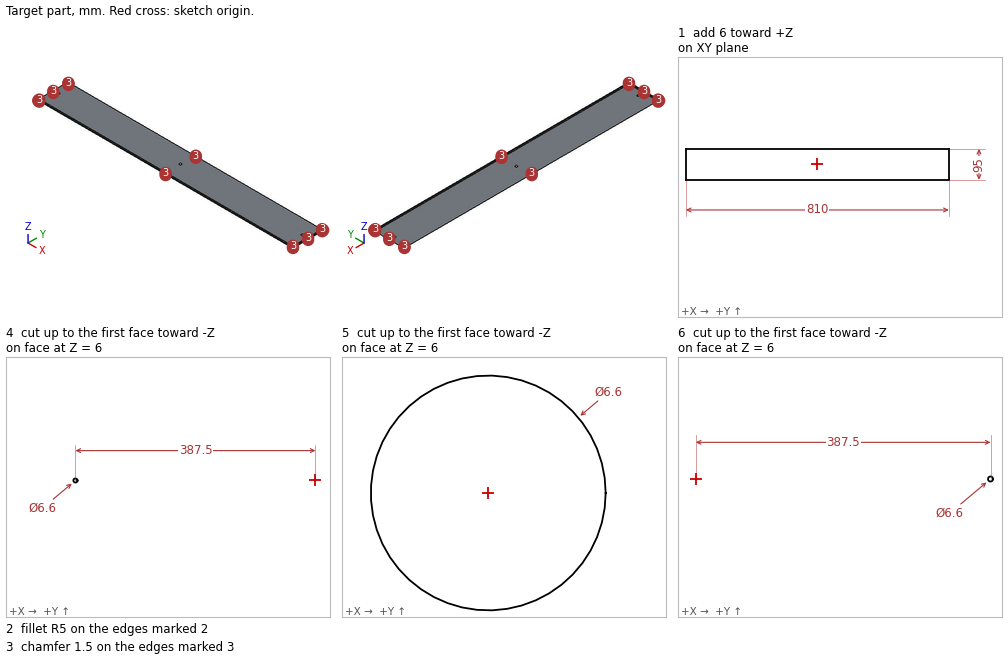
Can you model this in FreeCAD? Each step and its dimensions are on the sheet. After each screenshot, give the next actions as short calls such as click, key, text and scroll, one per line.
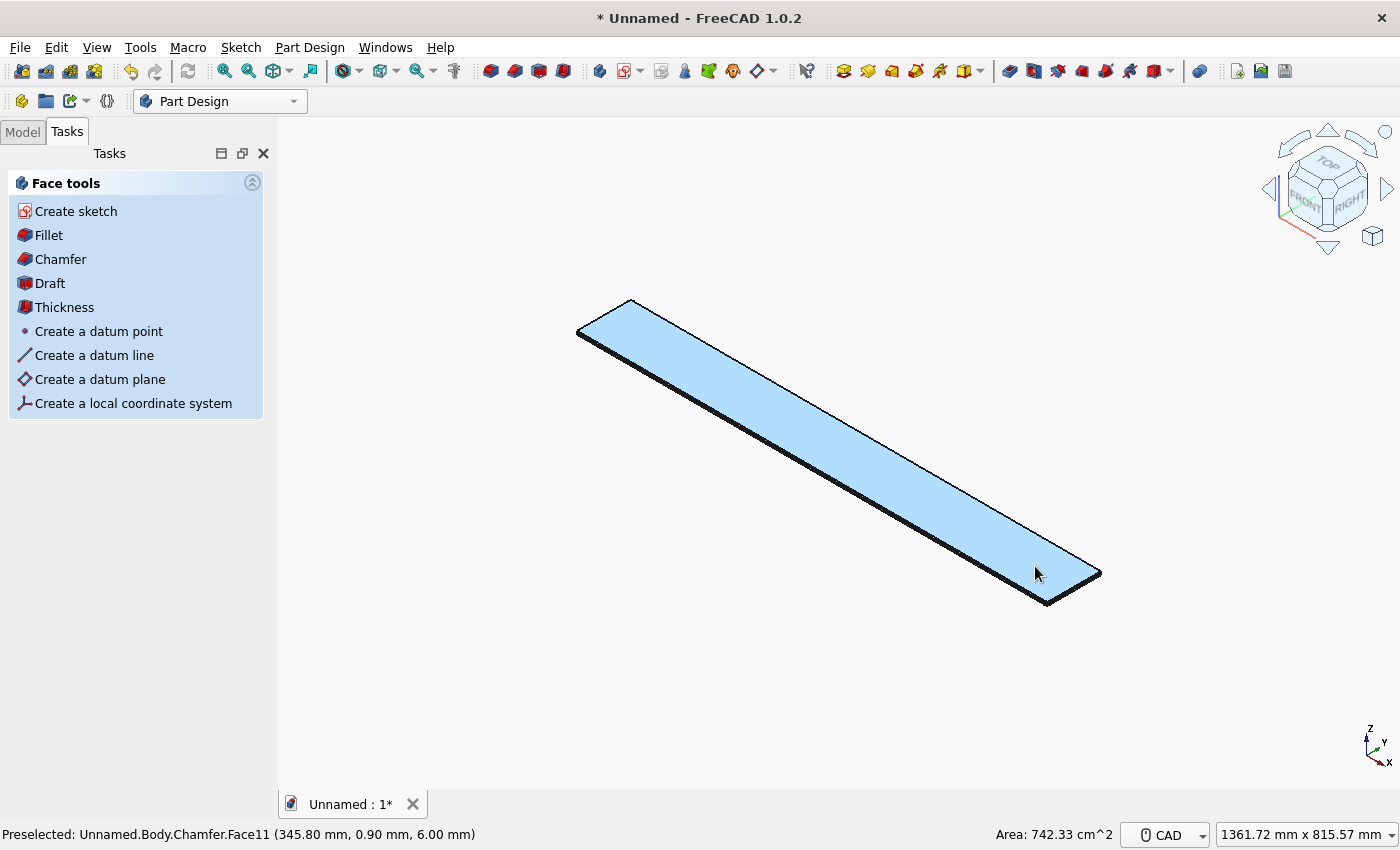
click(624, 72)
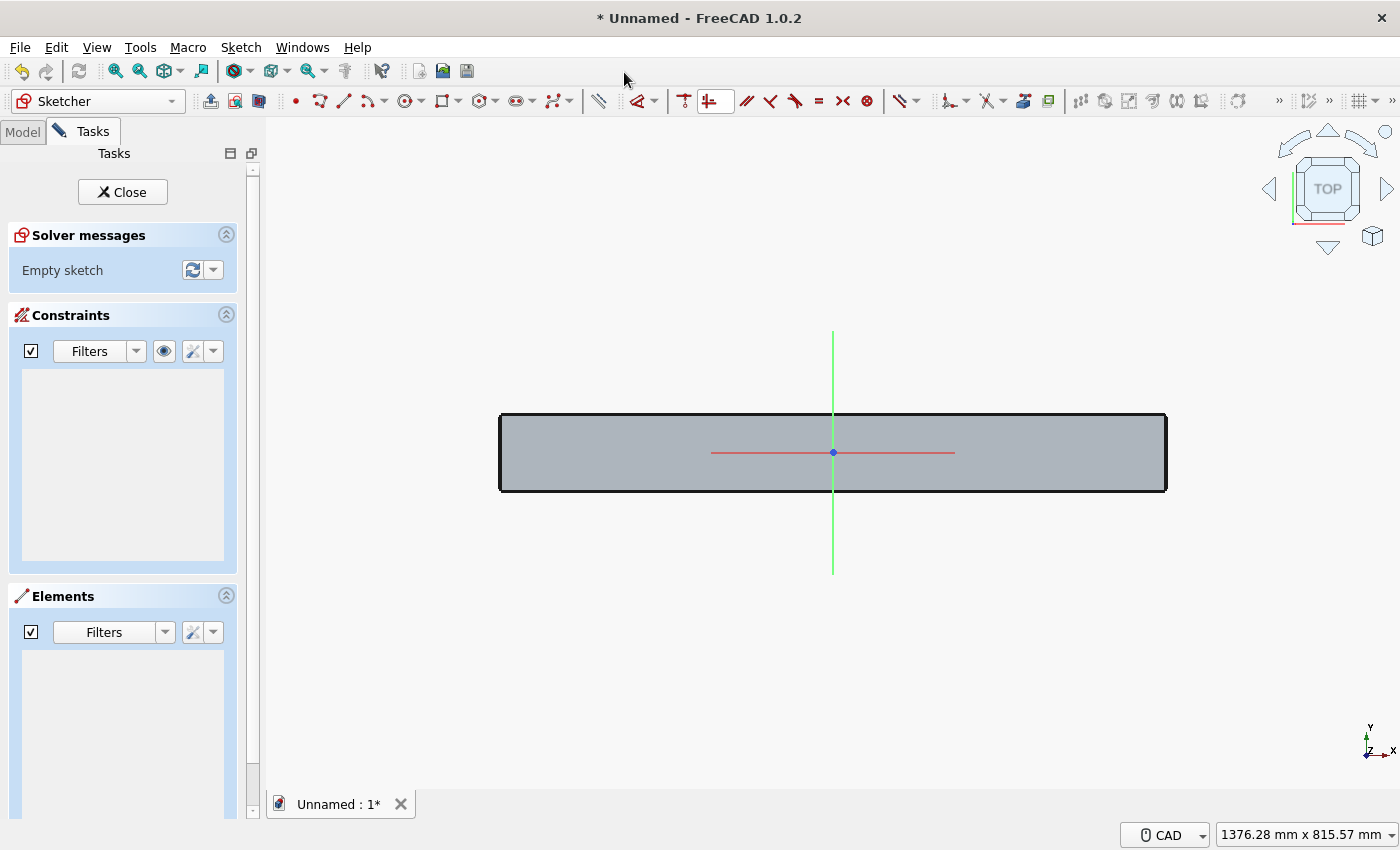
scroll(501, 453, up, 15)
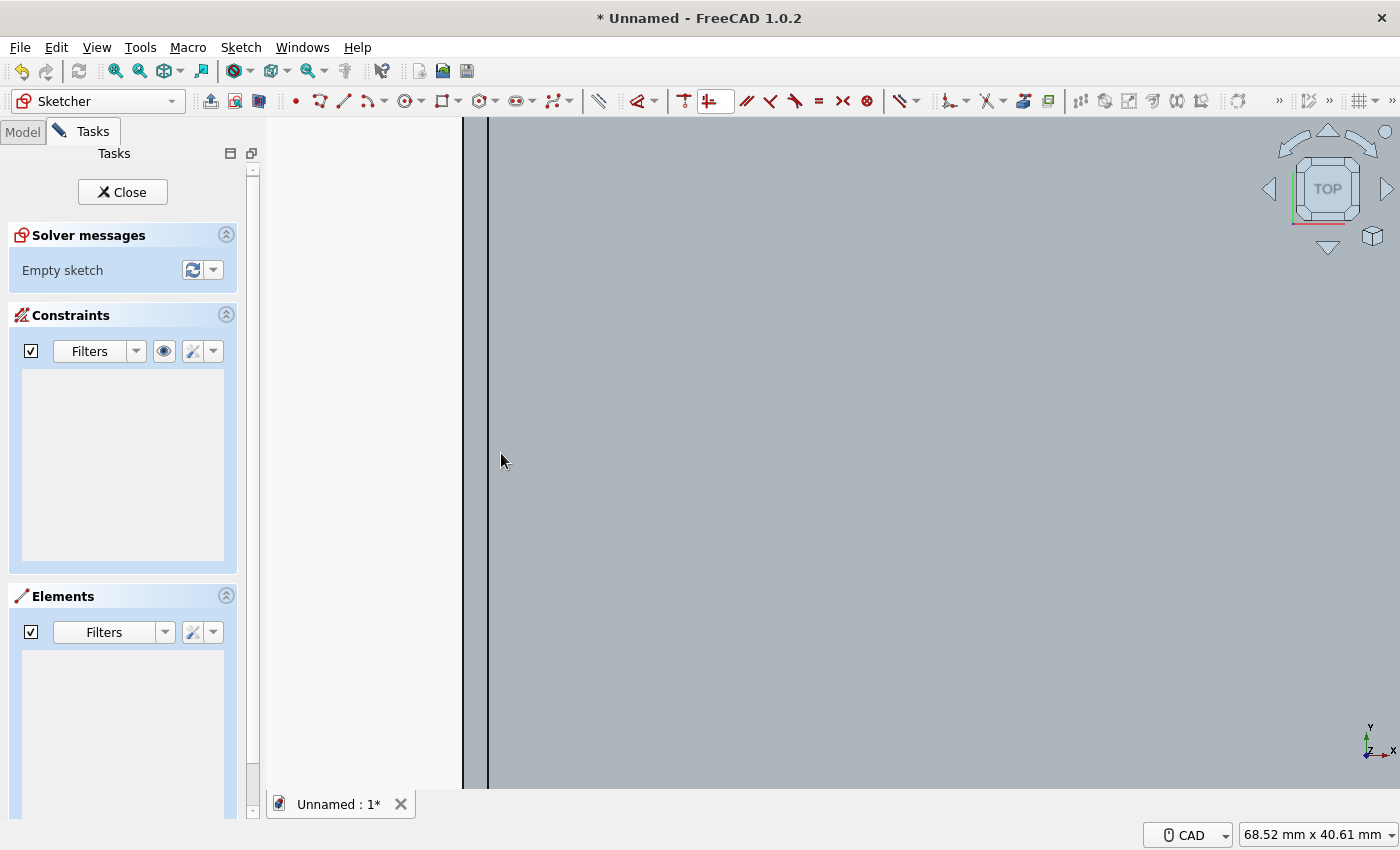
scroll(748, 440, up, 7)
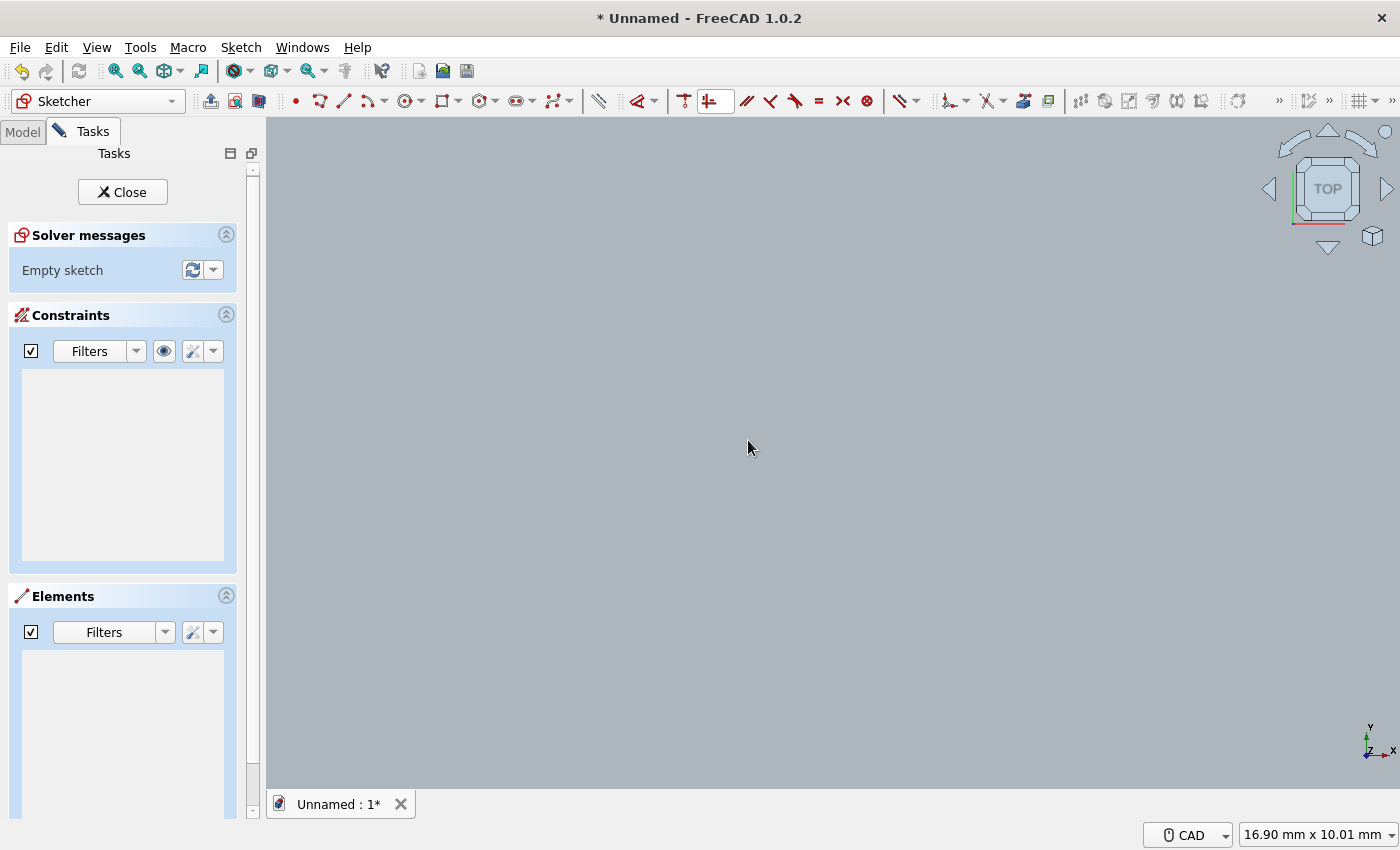
key(g)
key(c)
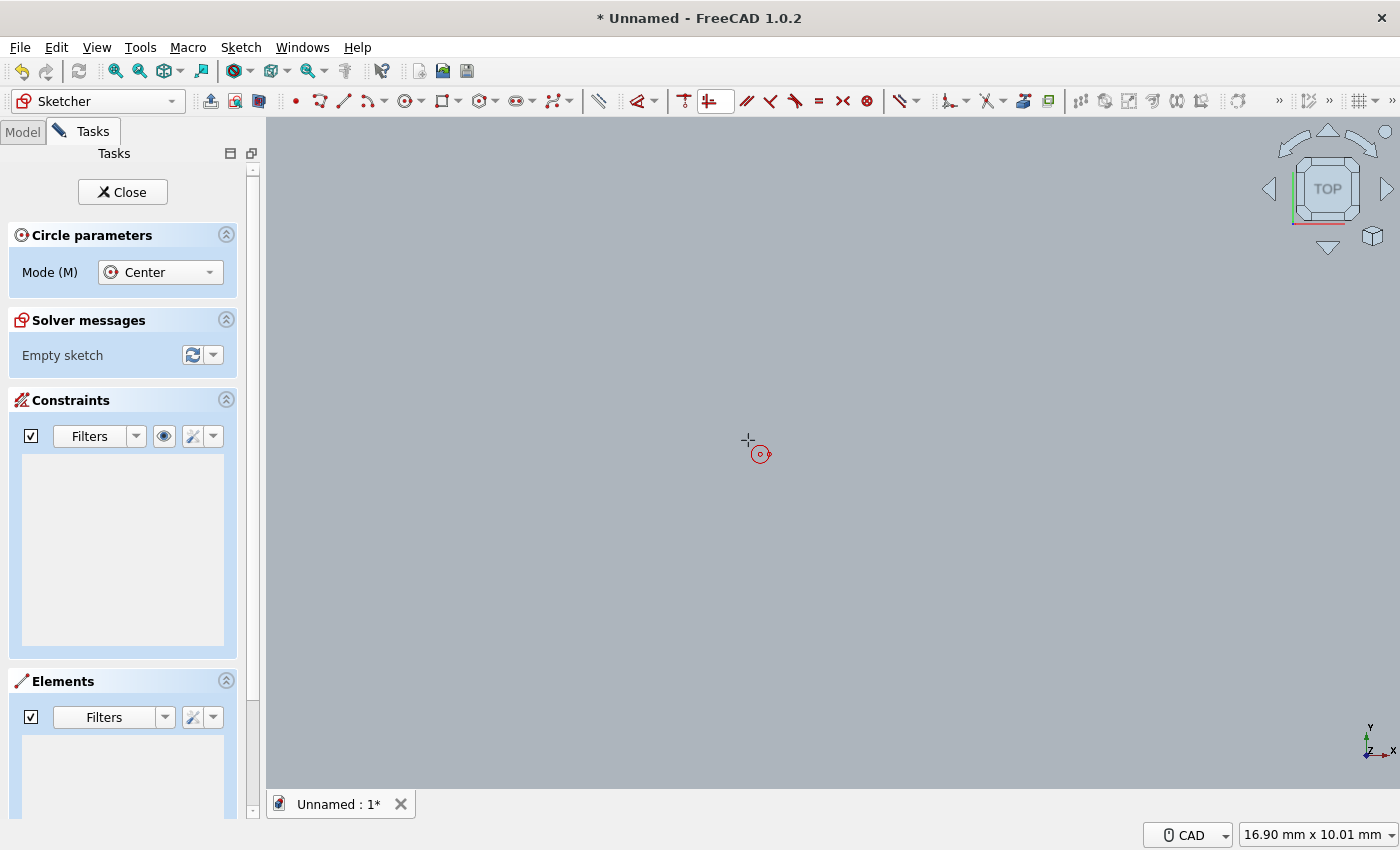
click(765, 452)
move(921, 296)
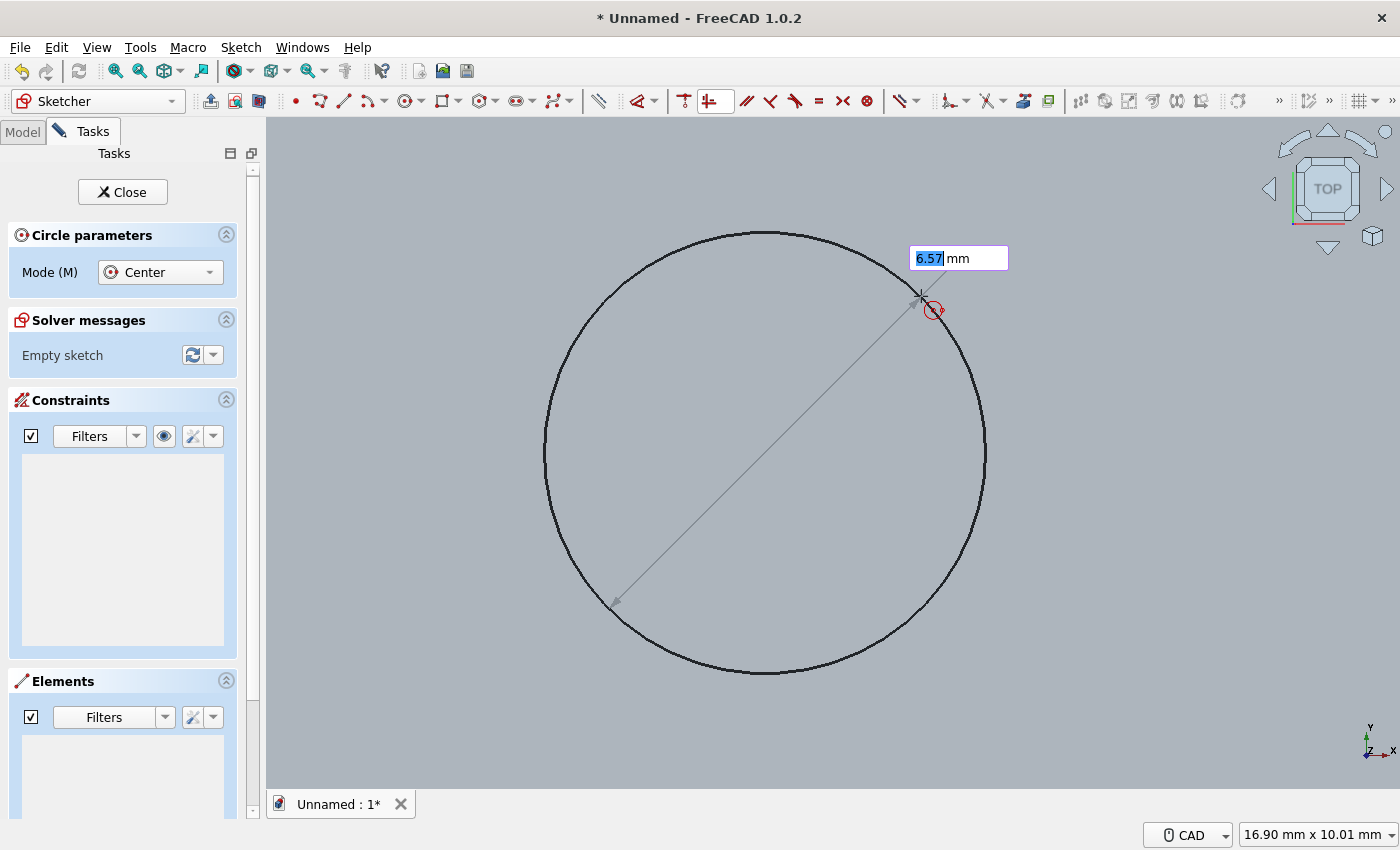
text(6.6)
key(Return)
key(Escape)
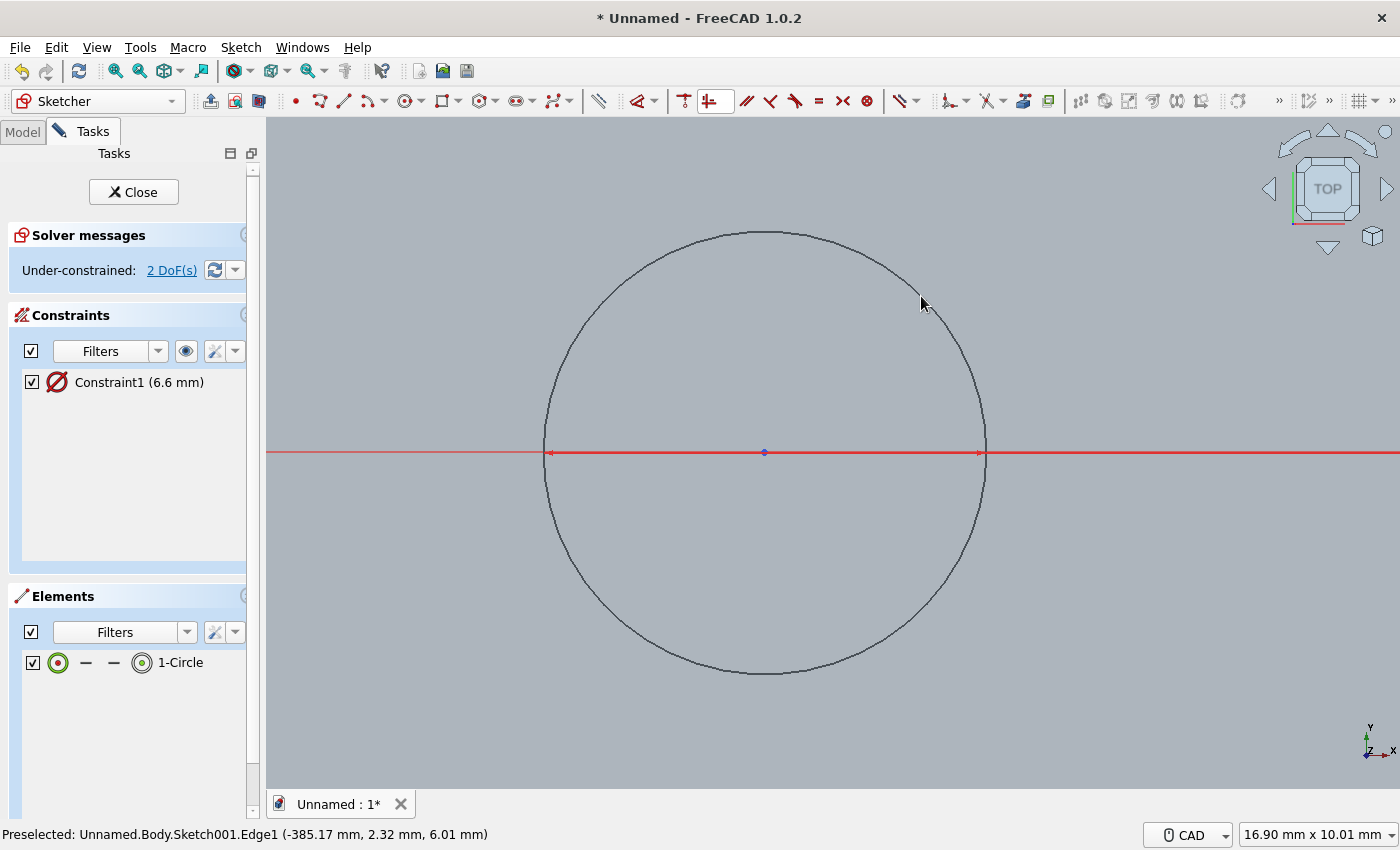
click(765, 453)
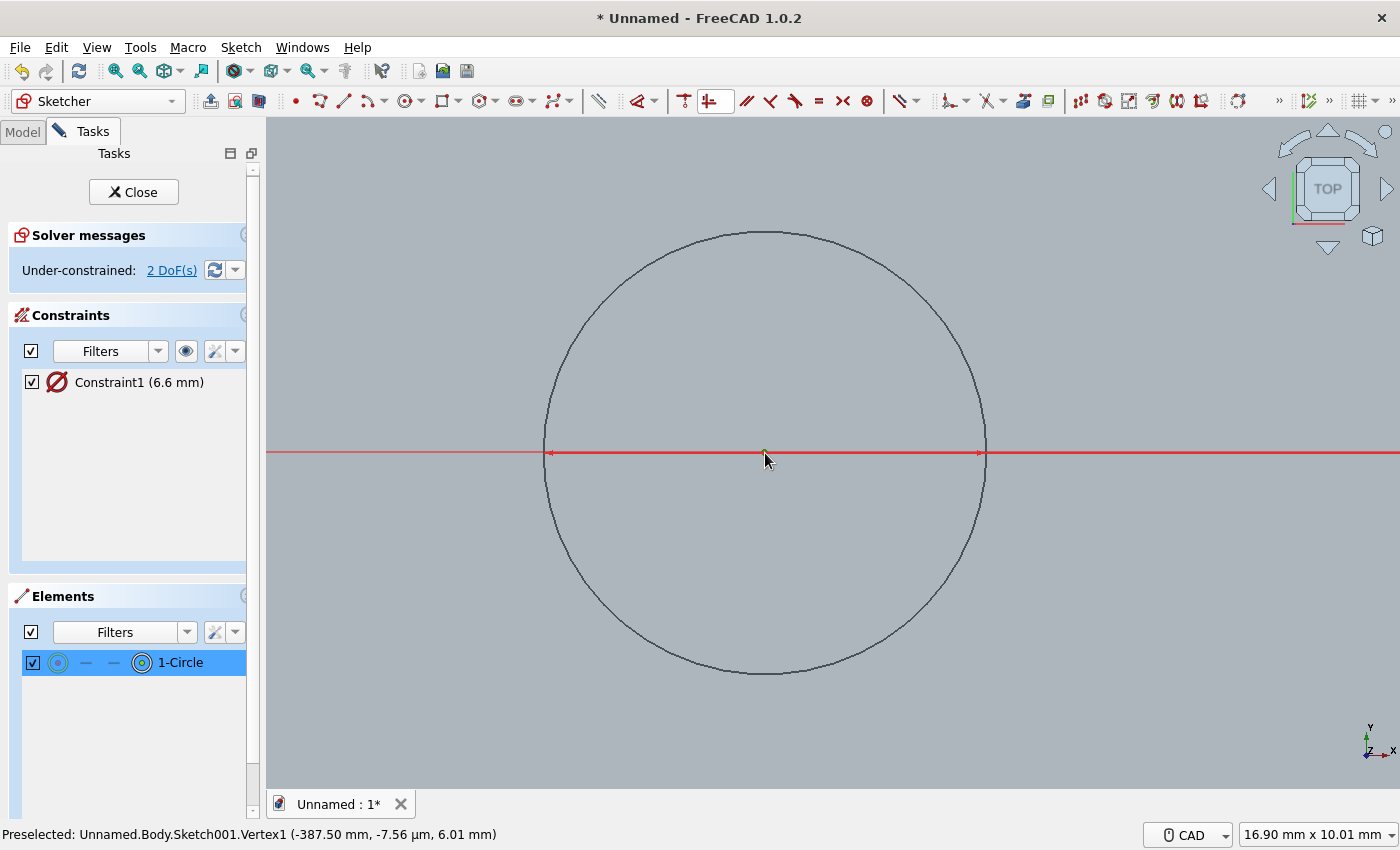
click(361, 452)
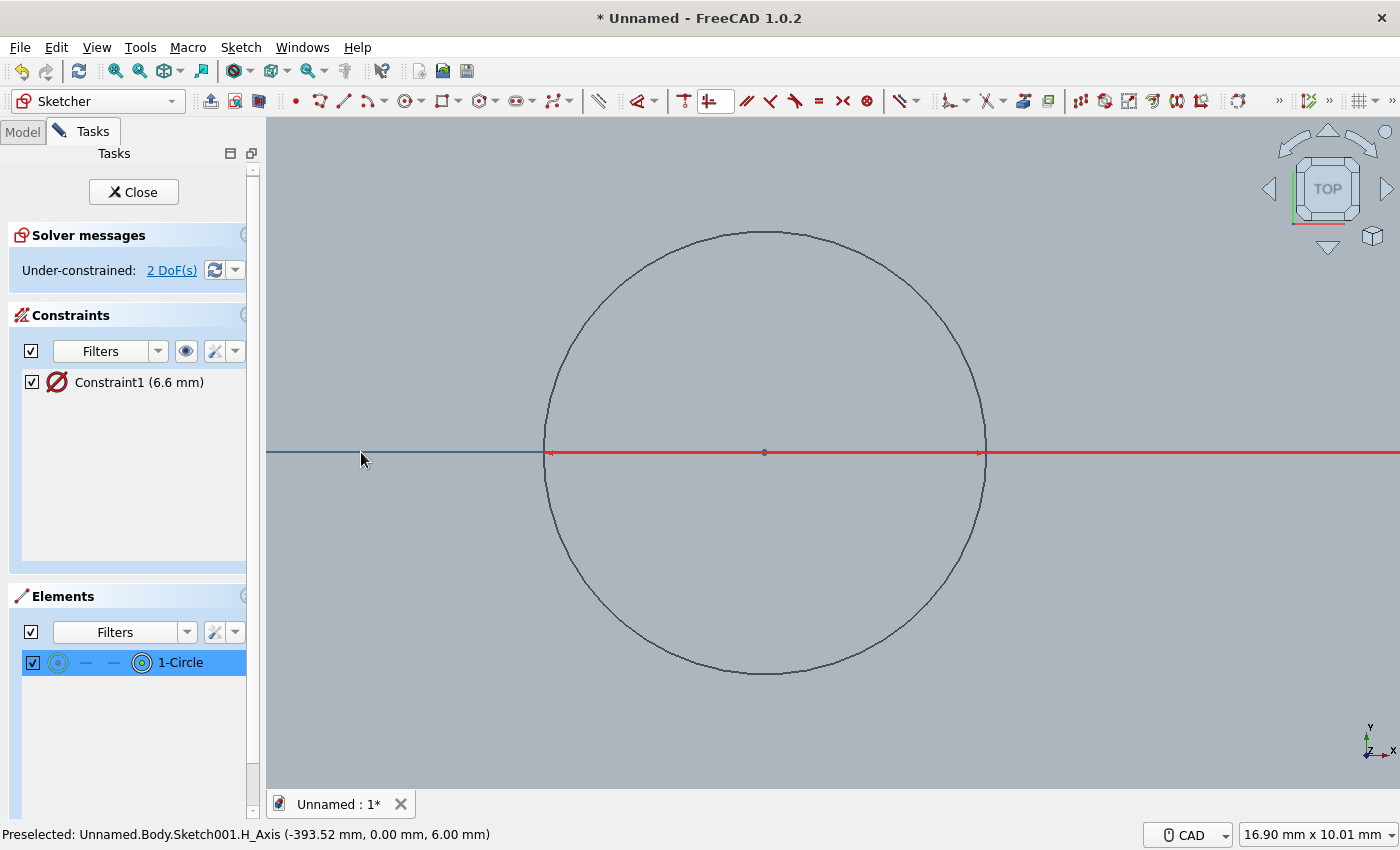
key(c)